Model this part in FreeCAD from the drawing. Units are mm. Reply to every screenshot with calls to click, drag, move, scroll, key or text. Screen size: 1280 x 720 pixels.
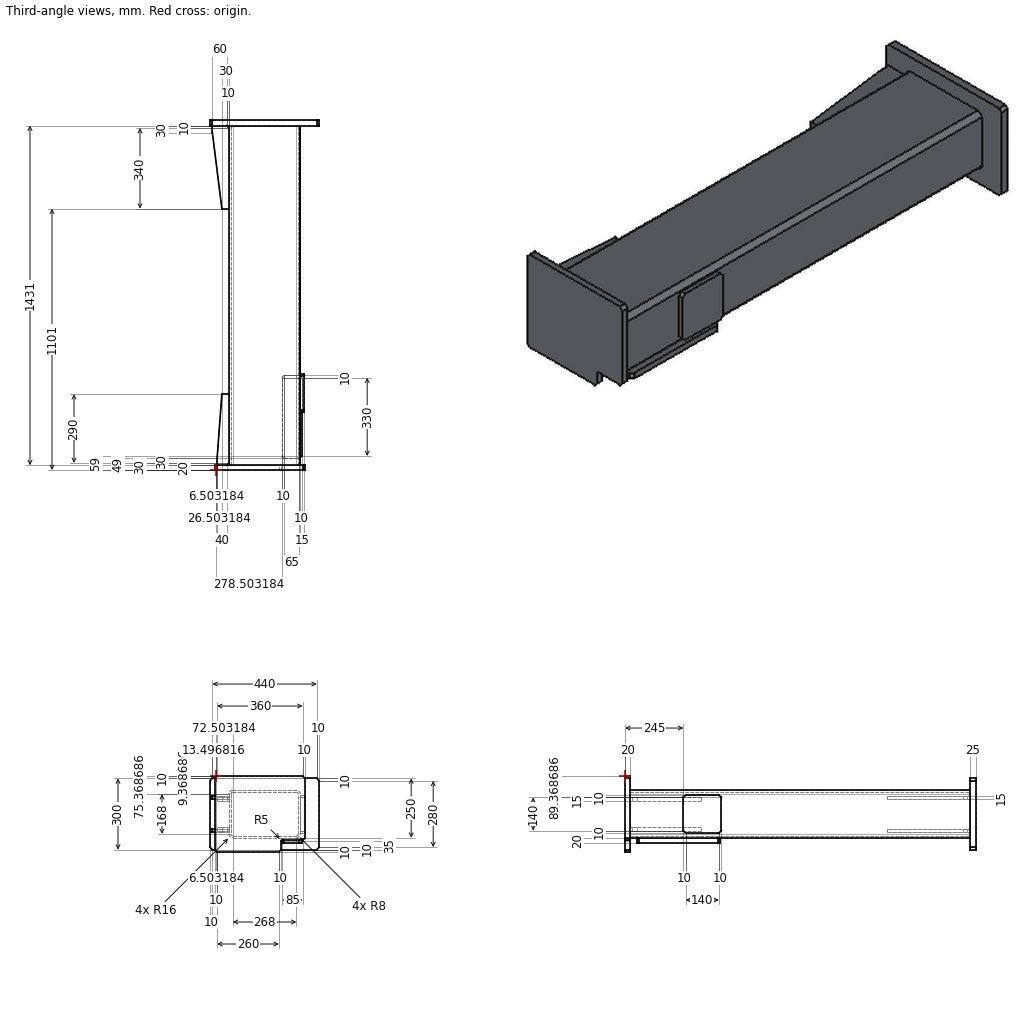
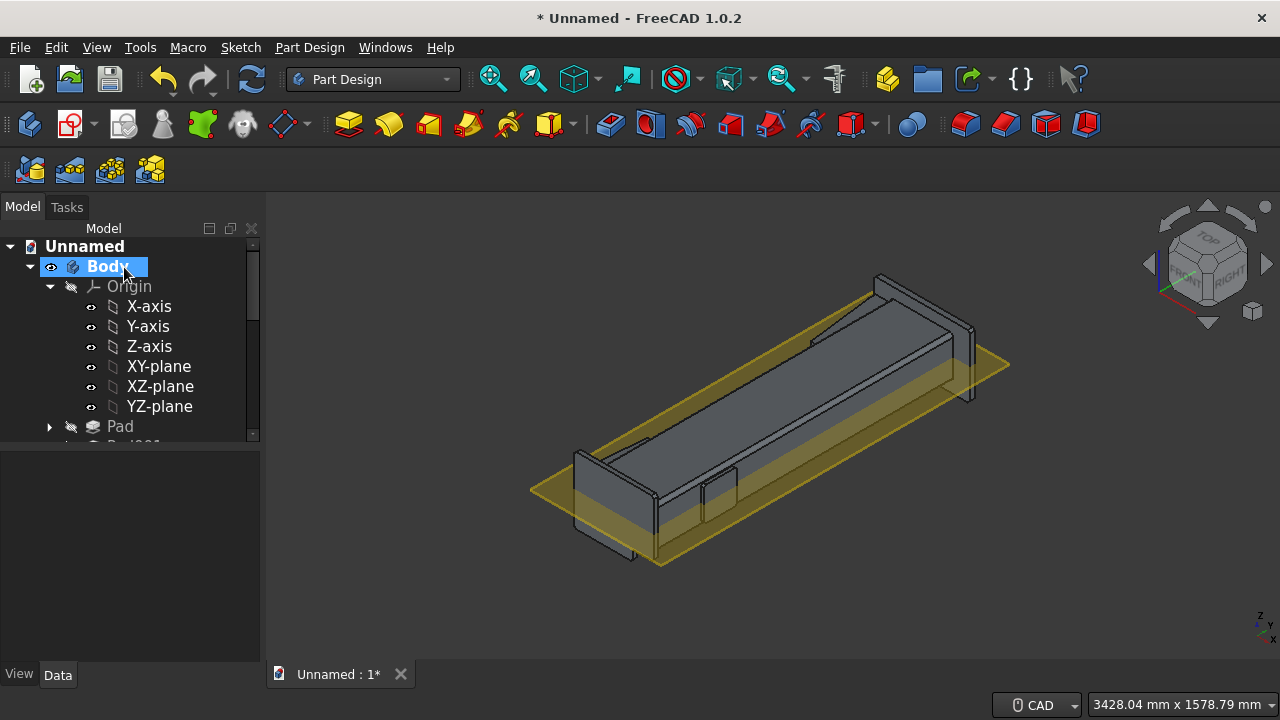
scroll(100, 342, down, 3)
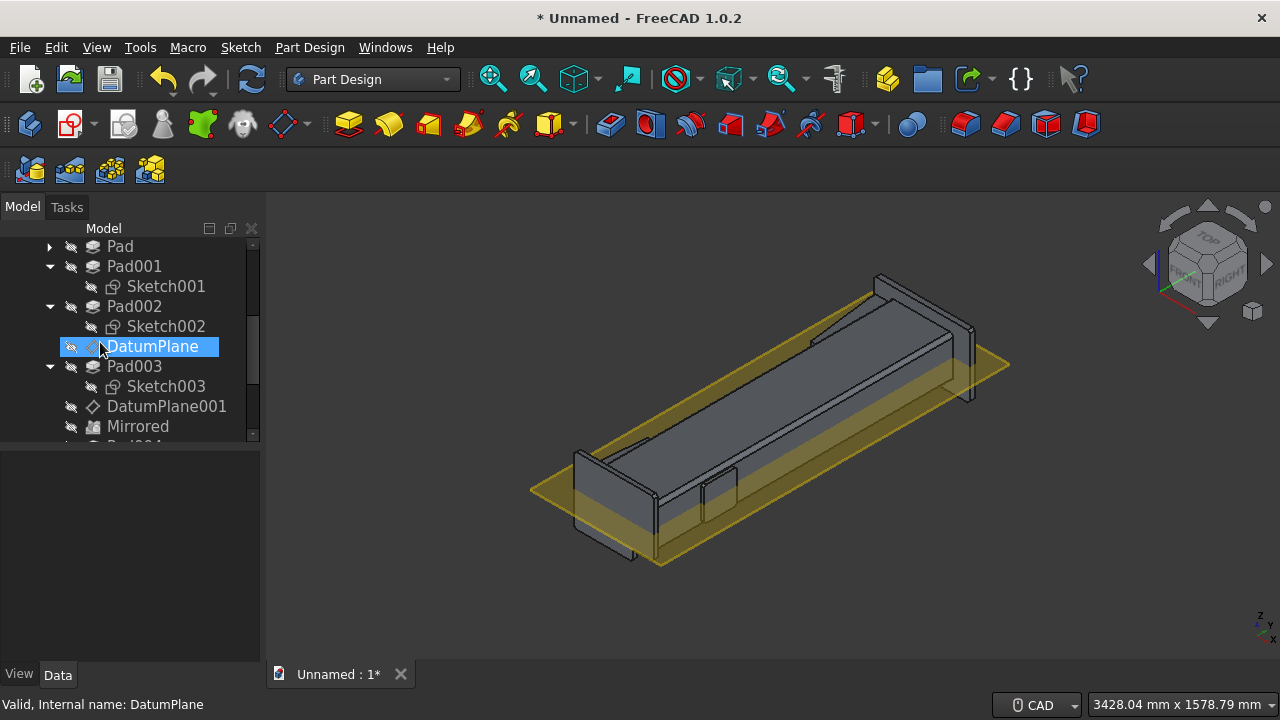
scroll(140, 342, up, 15)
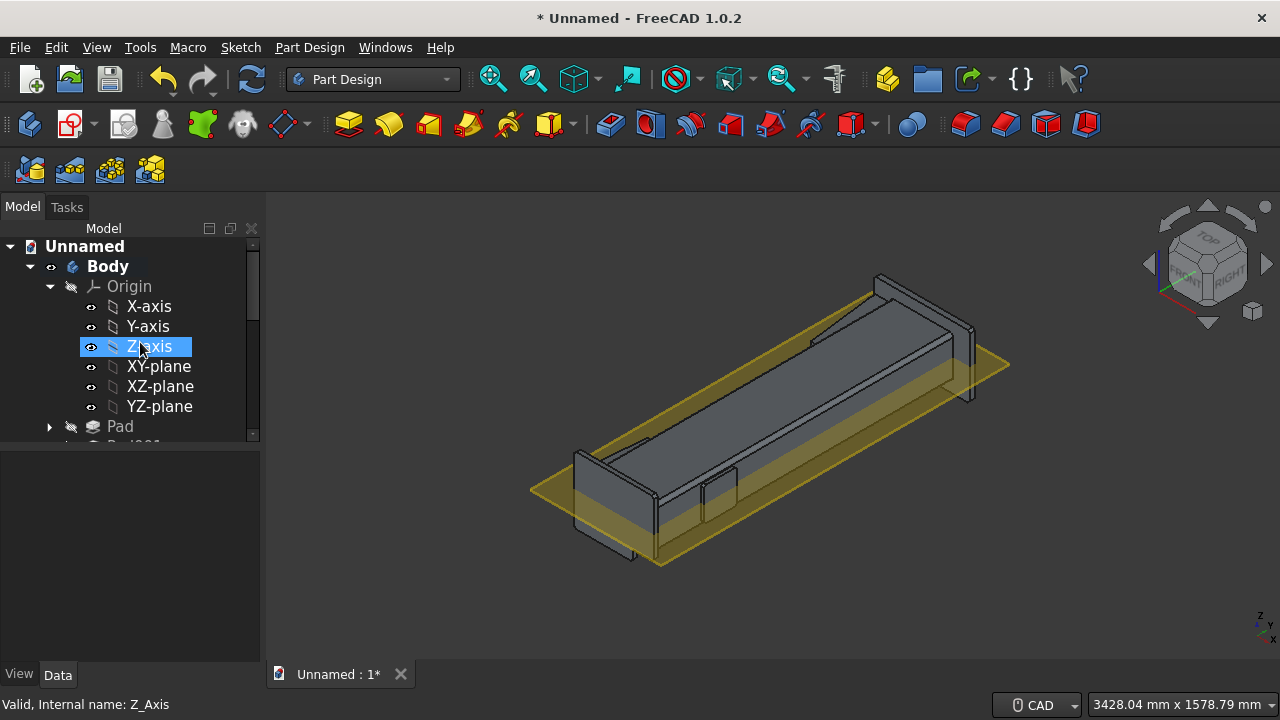
scroll(100, 342, down, 6)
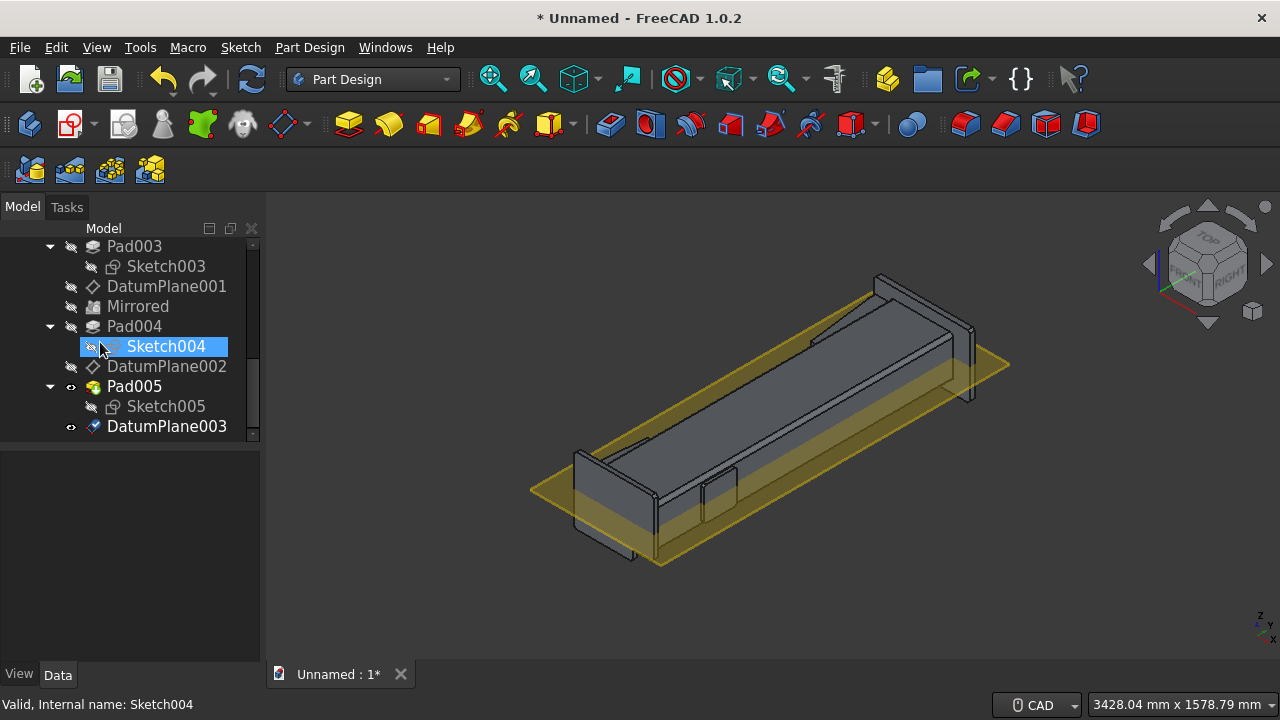
click(116, 387)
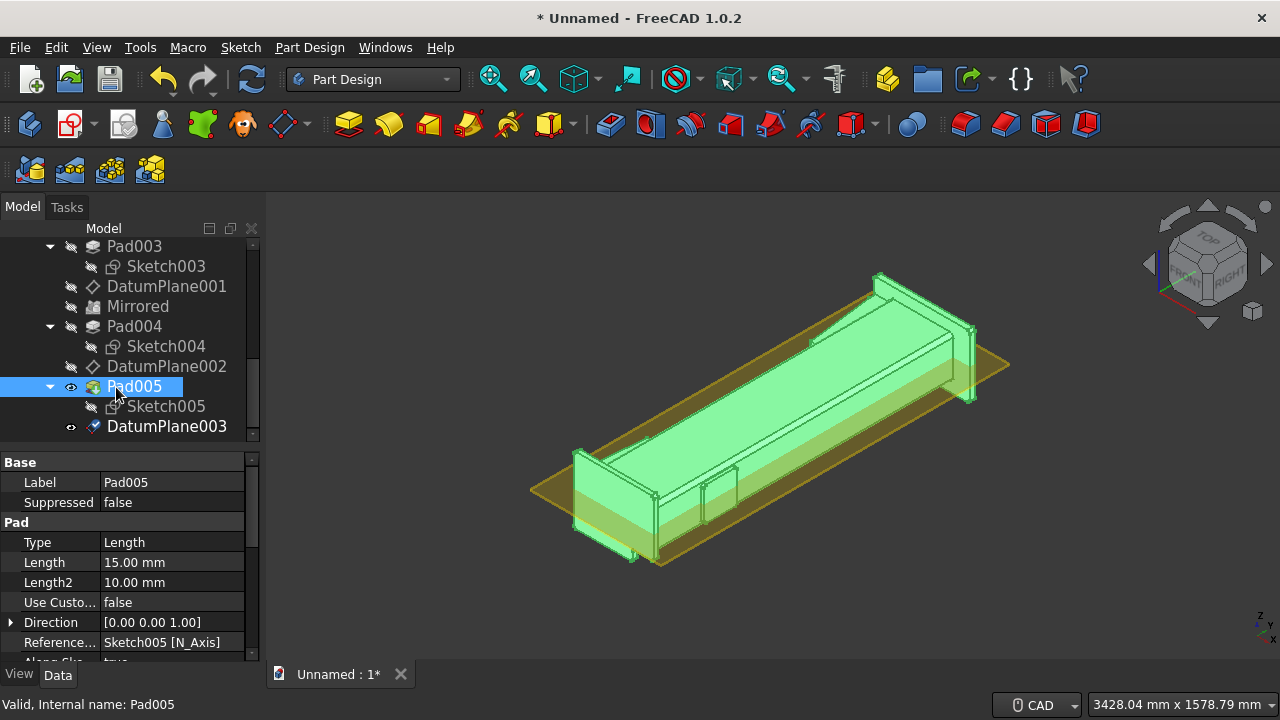
click(30, 170)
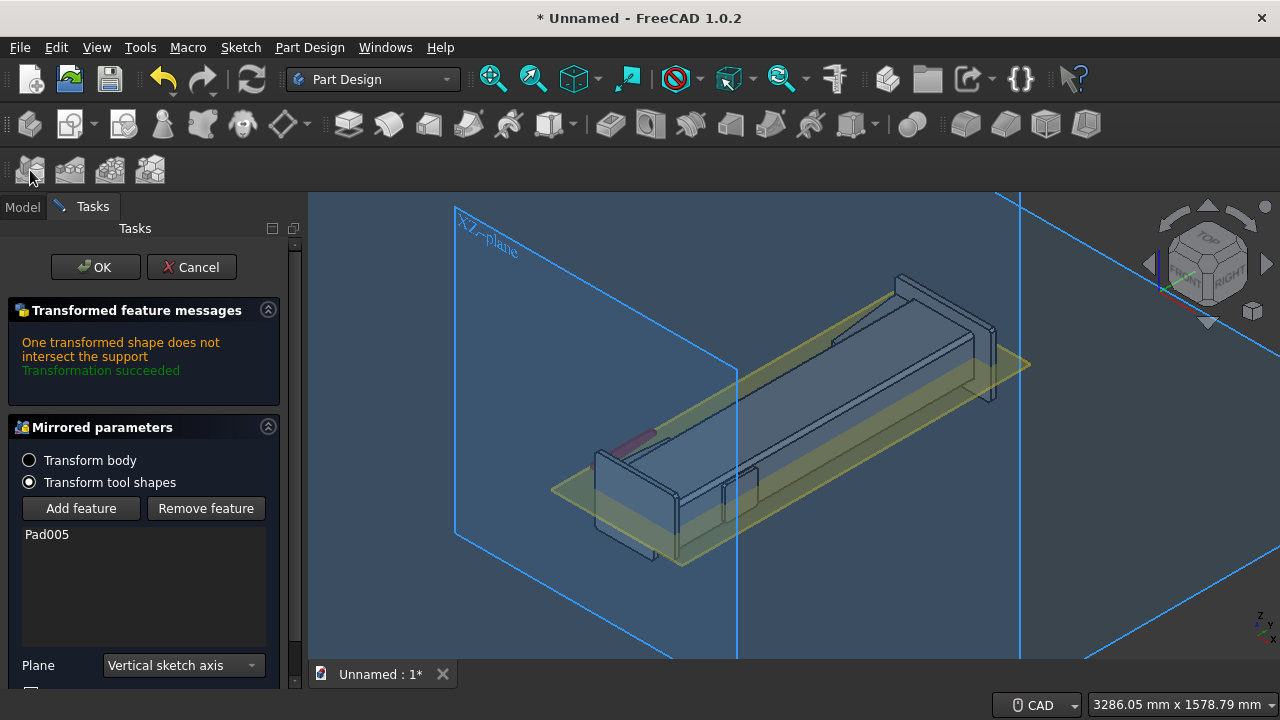
click(184, 666)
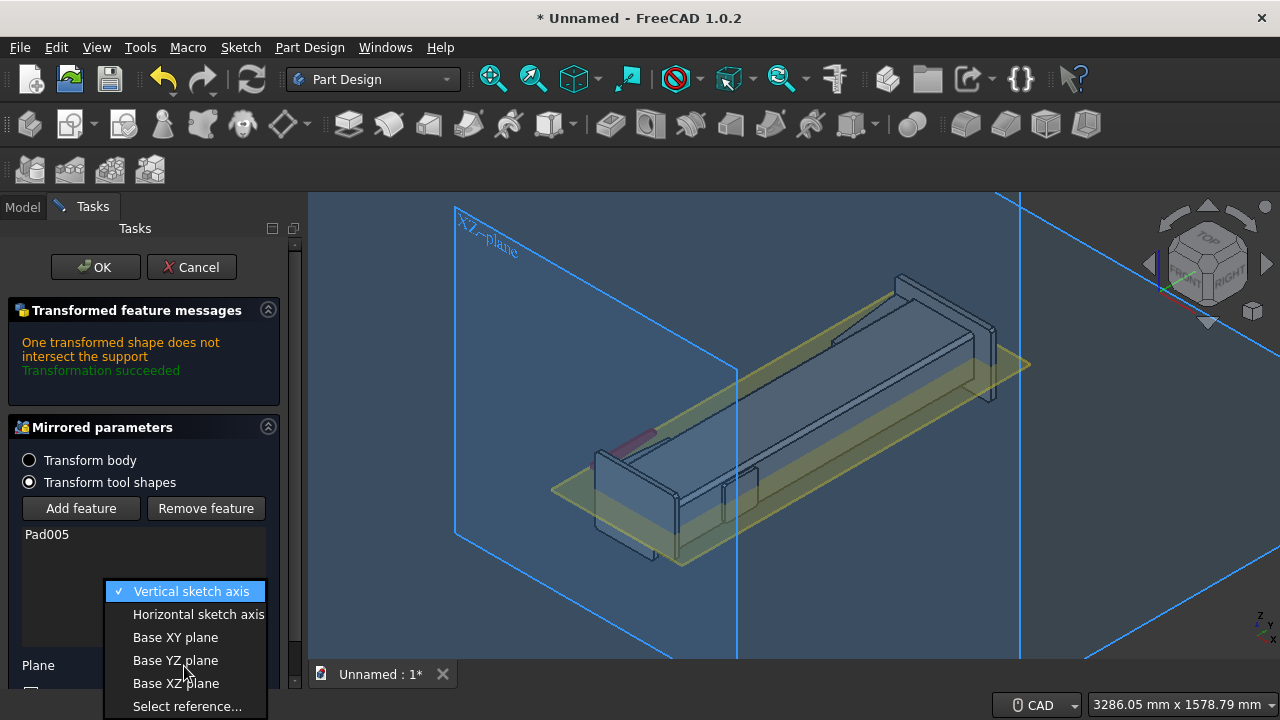
click(184, 706)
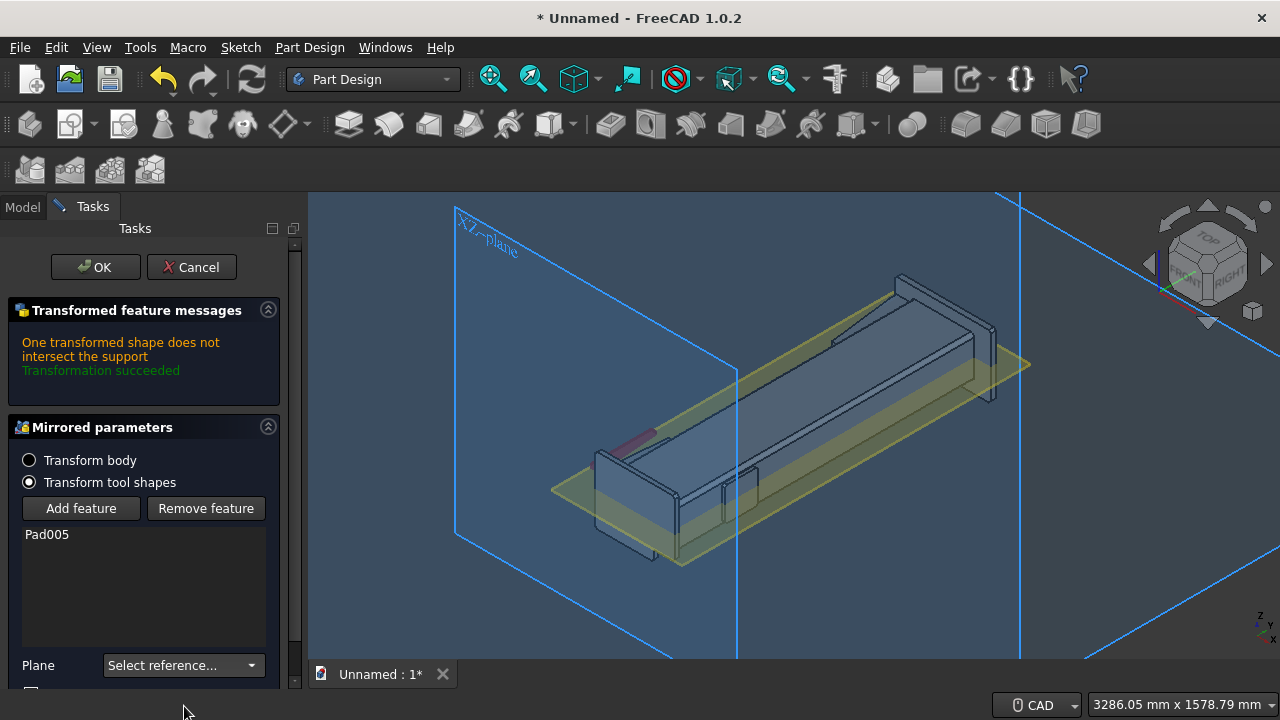
click(23, 206)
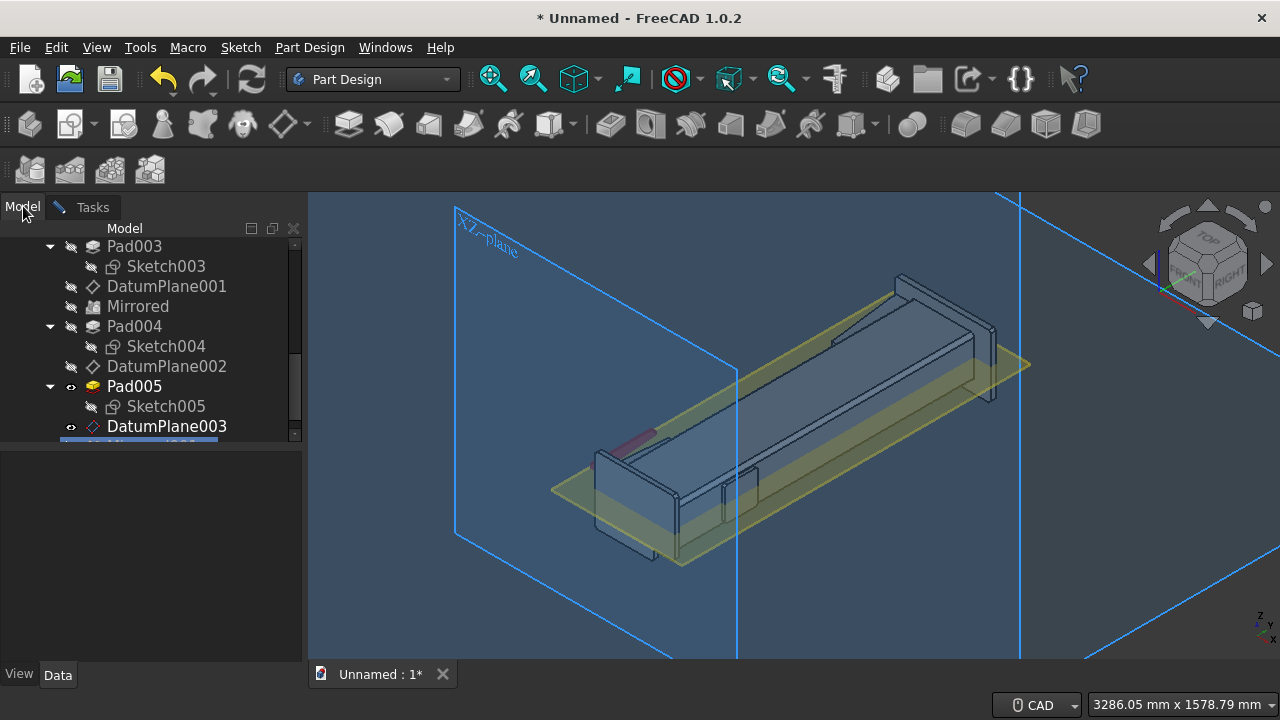
click(116, 427)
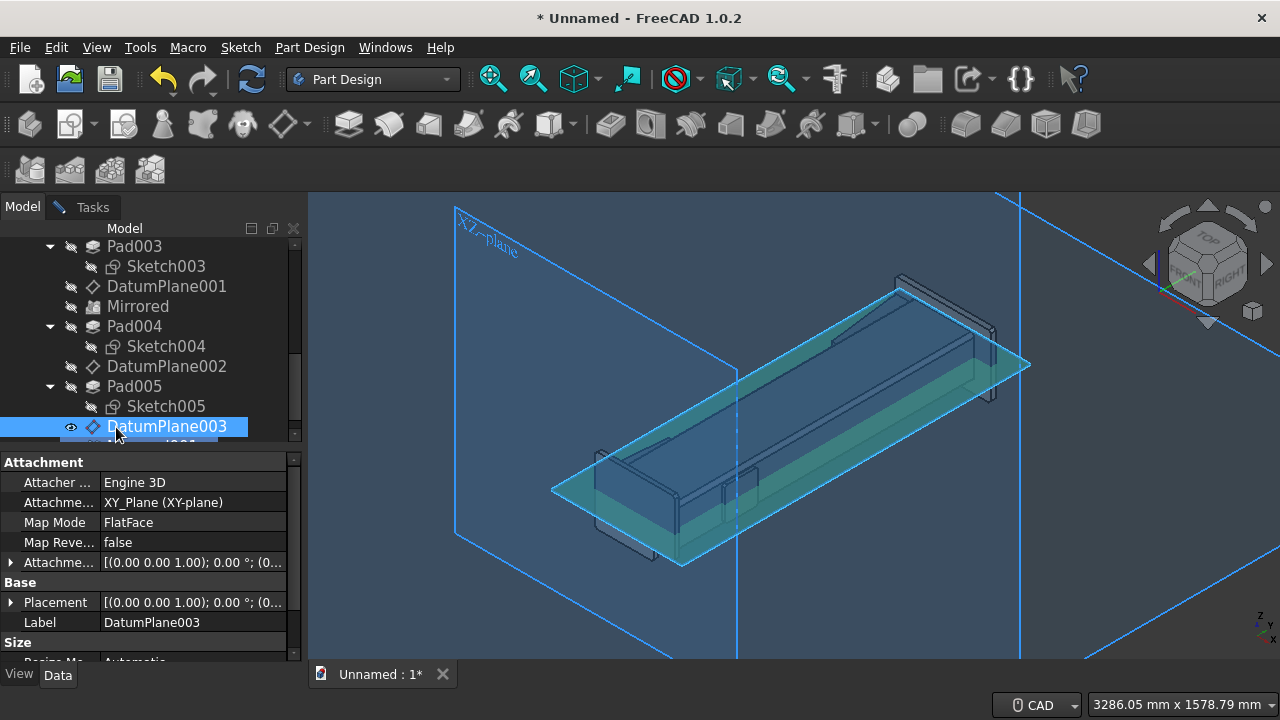
click(84, 206)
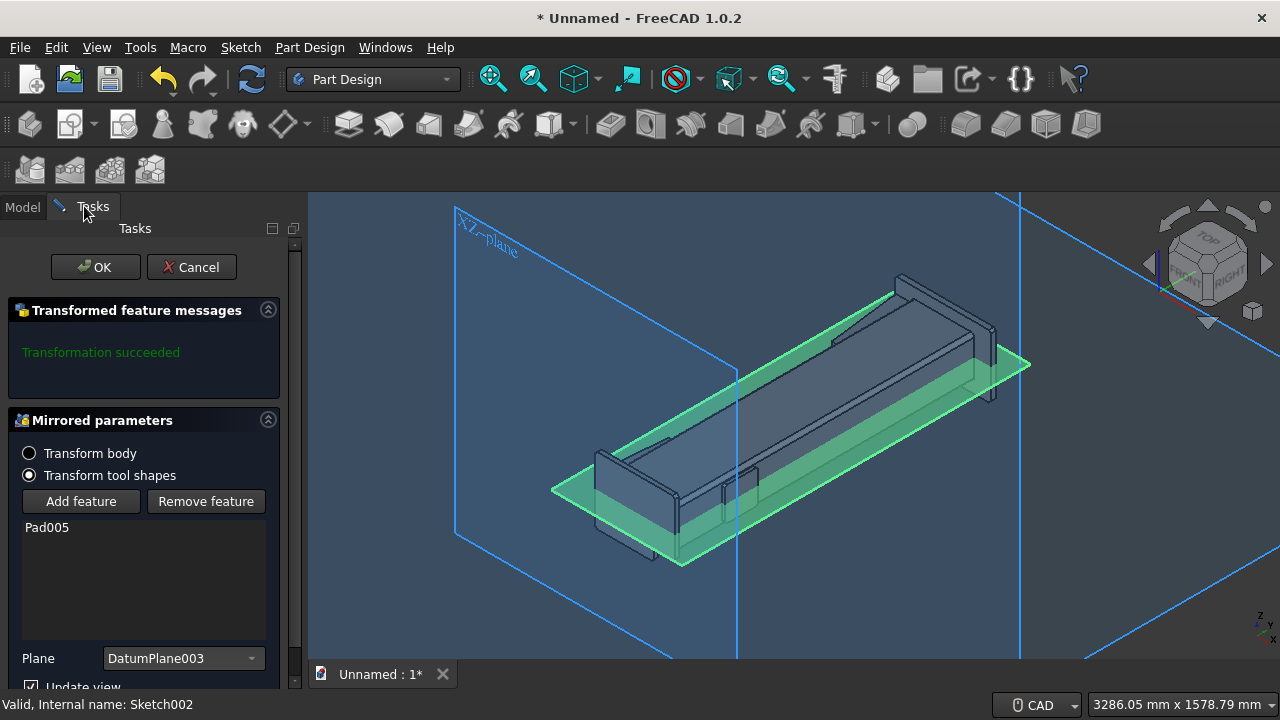
click(96, 267)